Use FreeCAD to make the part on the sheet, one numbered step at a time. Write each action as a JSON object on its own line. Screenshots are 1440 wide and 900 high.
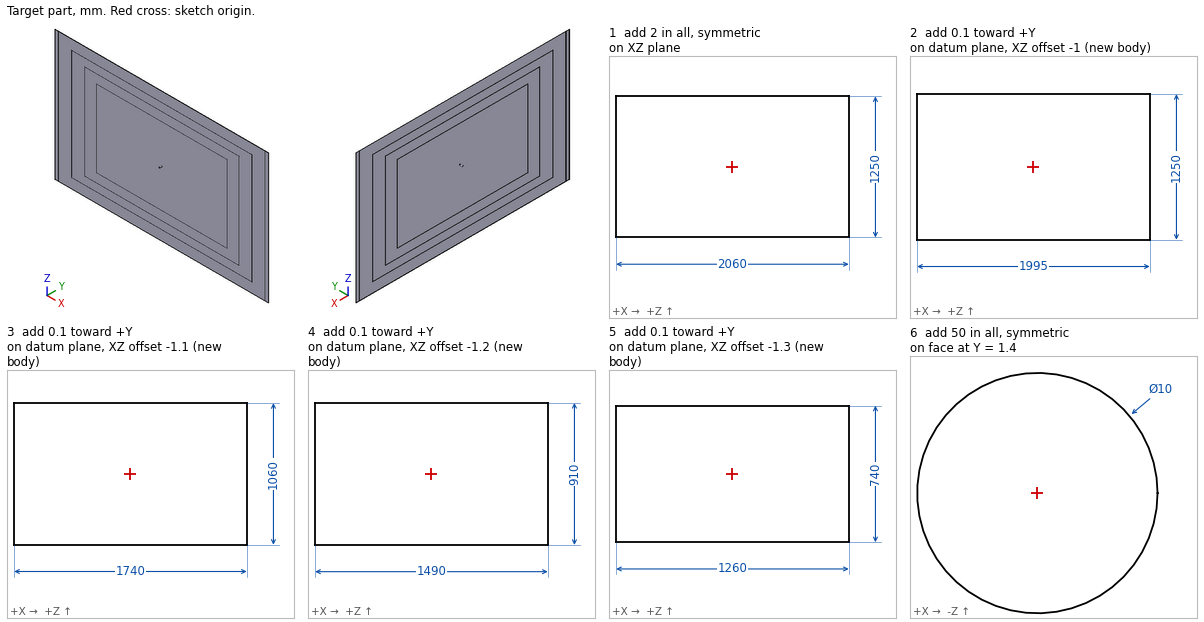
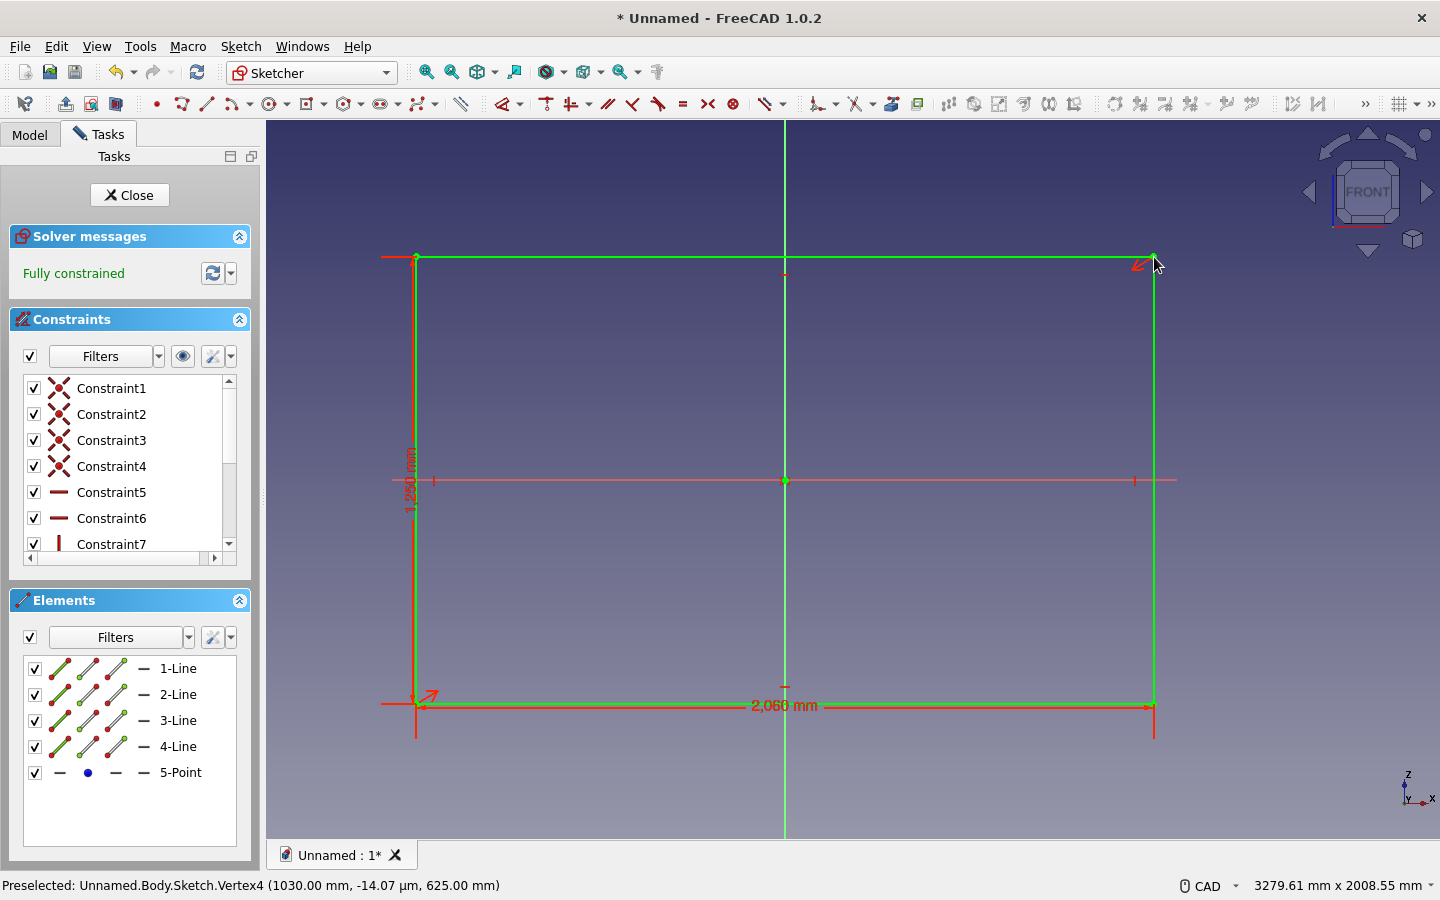
{"action": "left_click", "coordinate": [130, 195]}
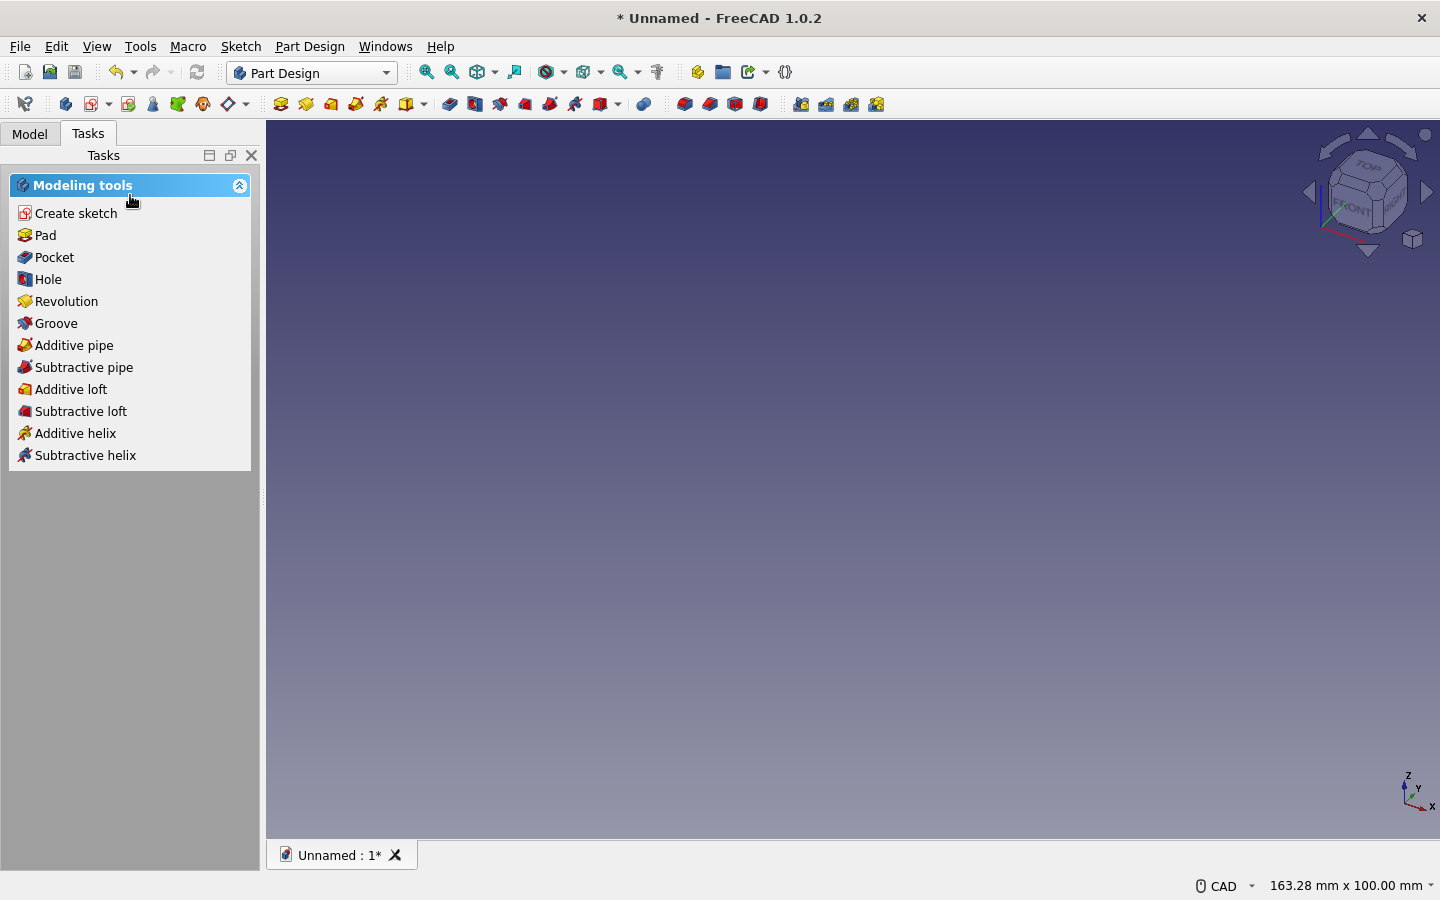
{"action": "left_click", "coordinate": [281, 104]}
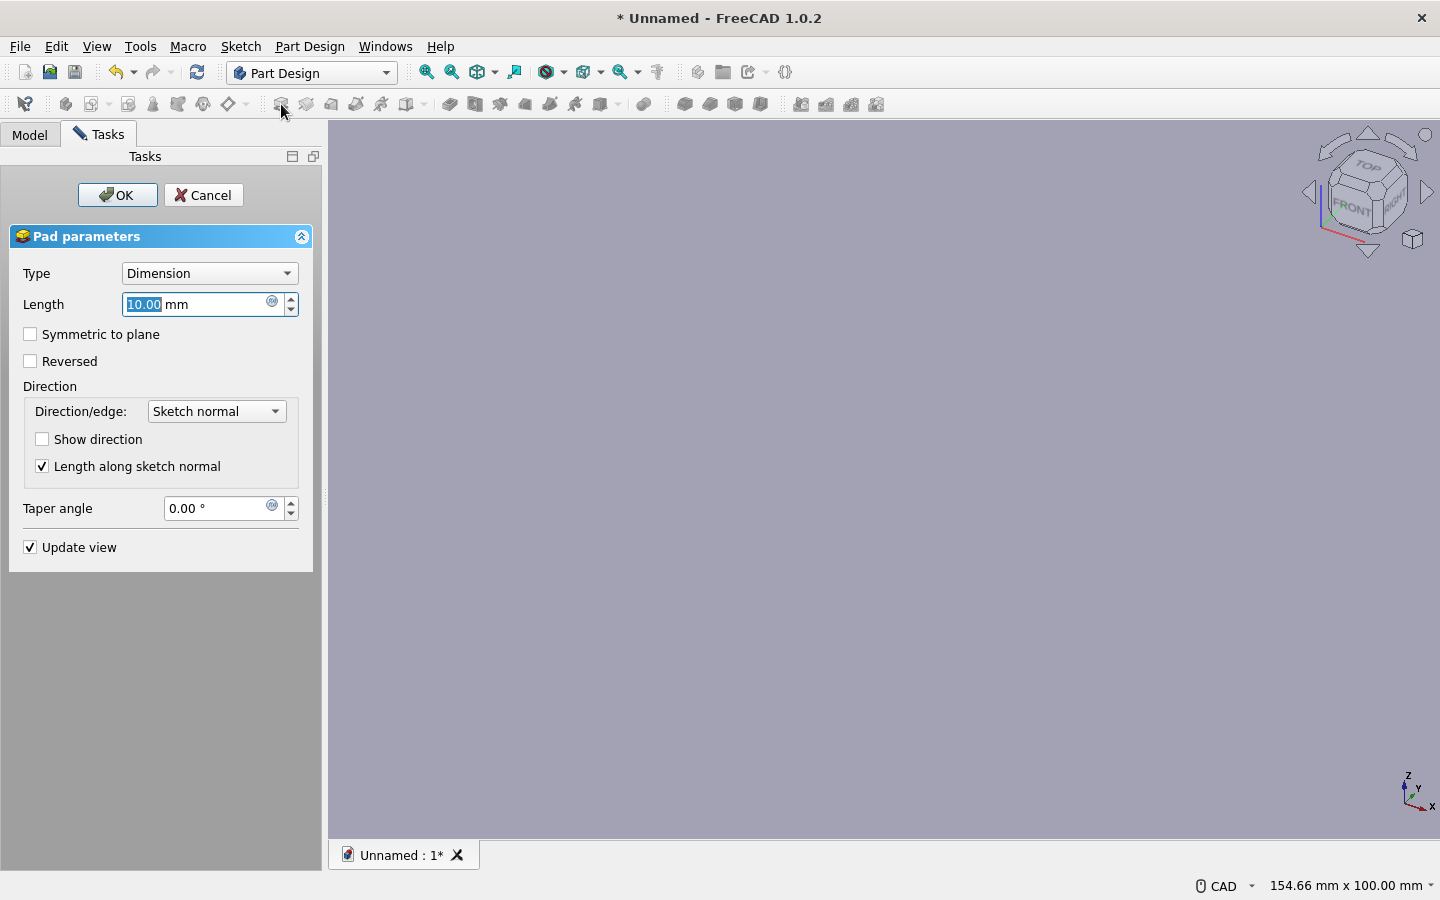
{"action": "type", "text": "2"}
{"action": "key", "text": "Tab"}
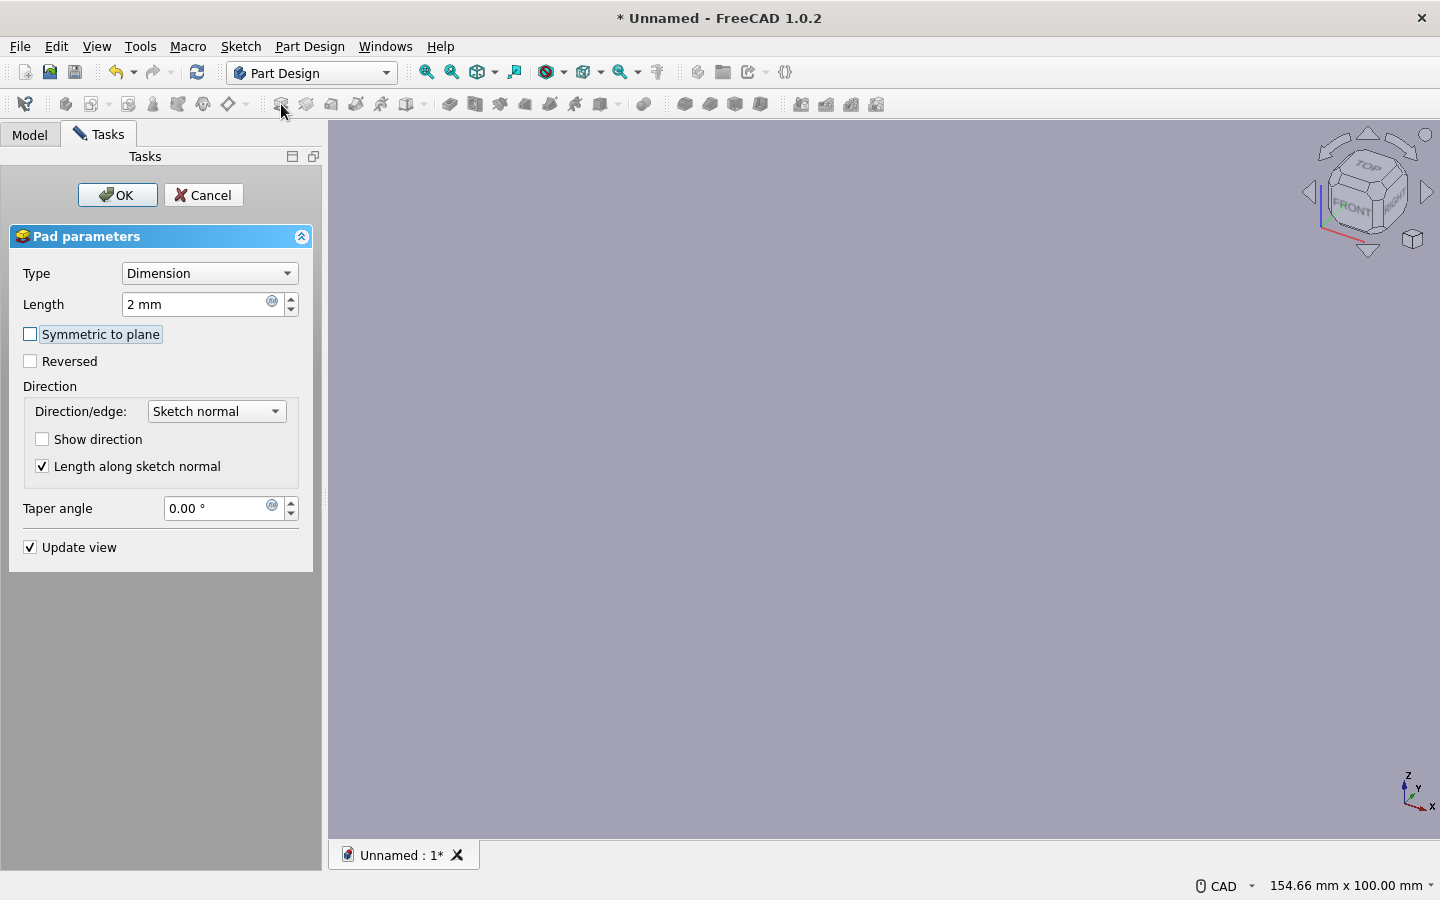
{"action": "left_click", "coordinate": [31, 334]}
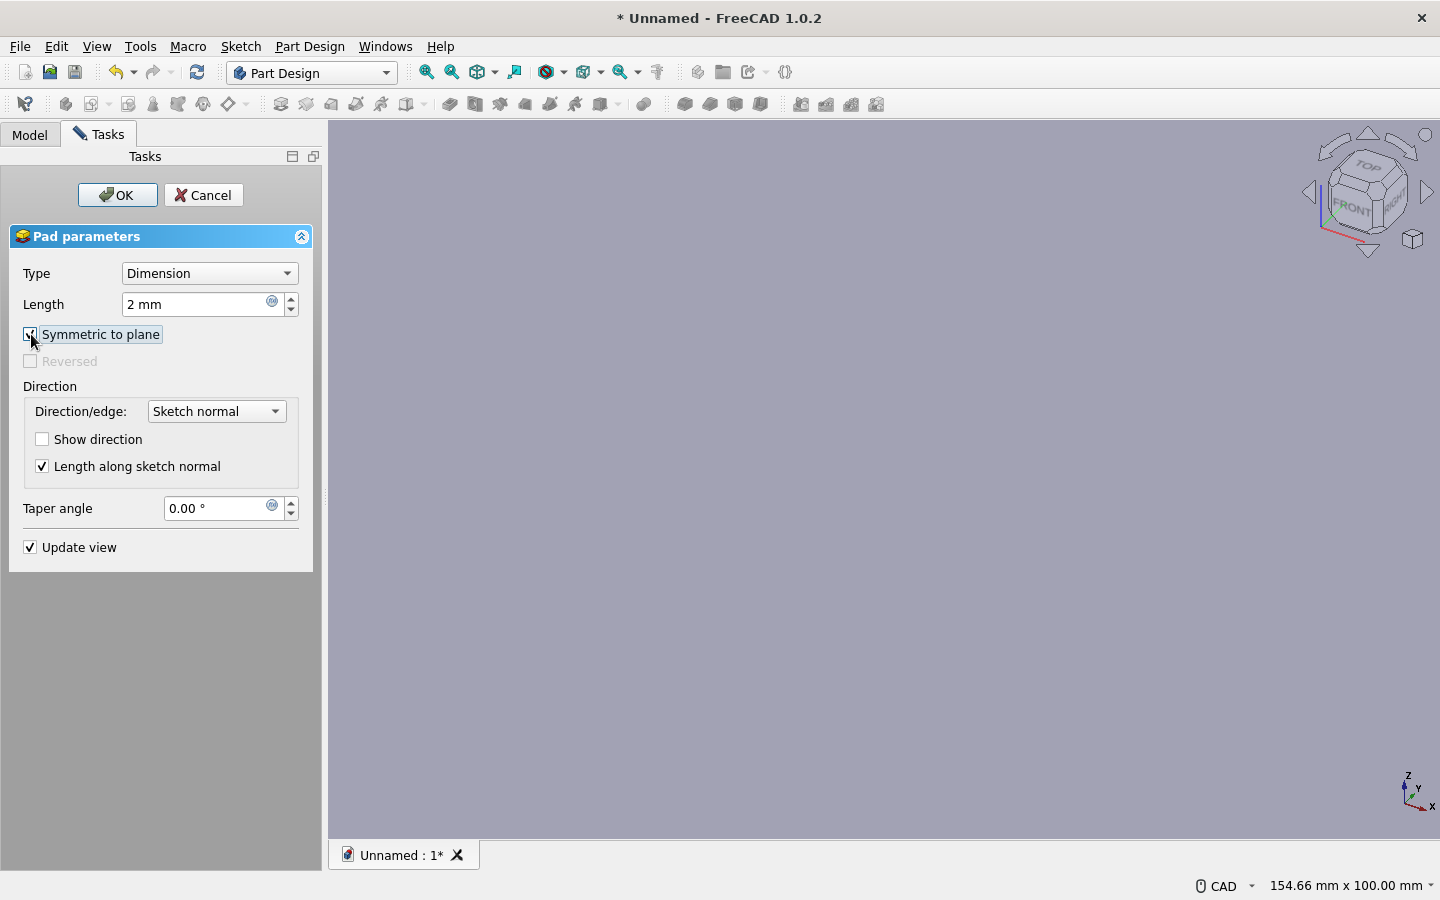
{"action": "left_click", "coordinate": [118, 195]}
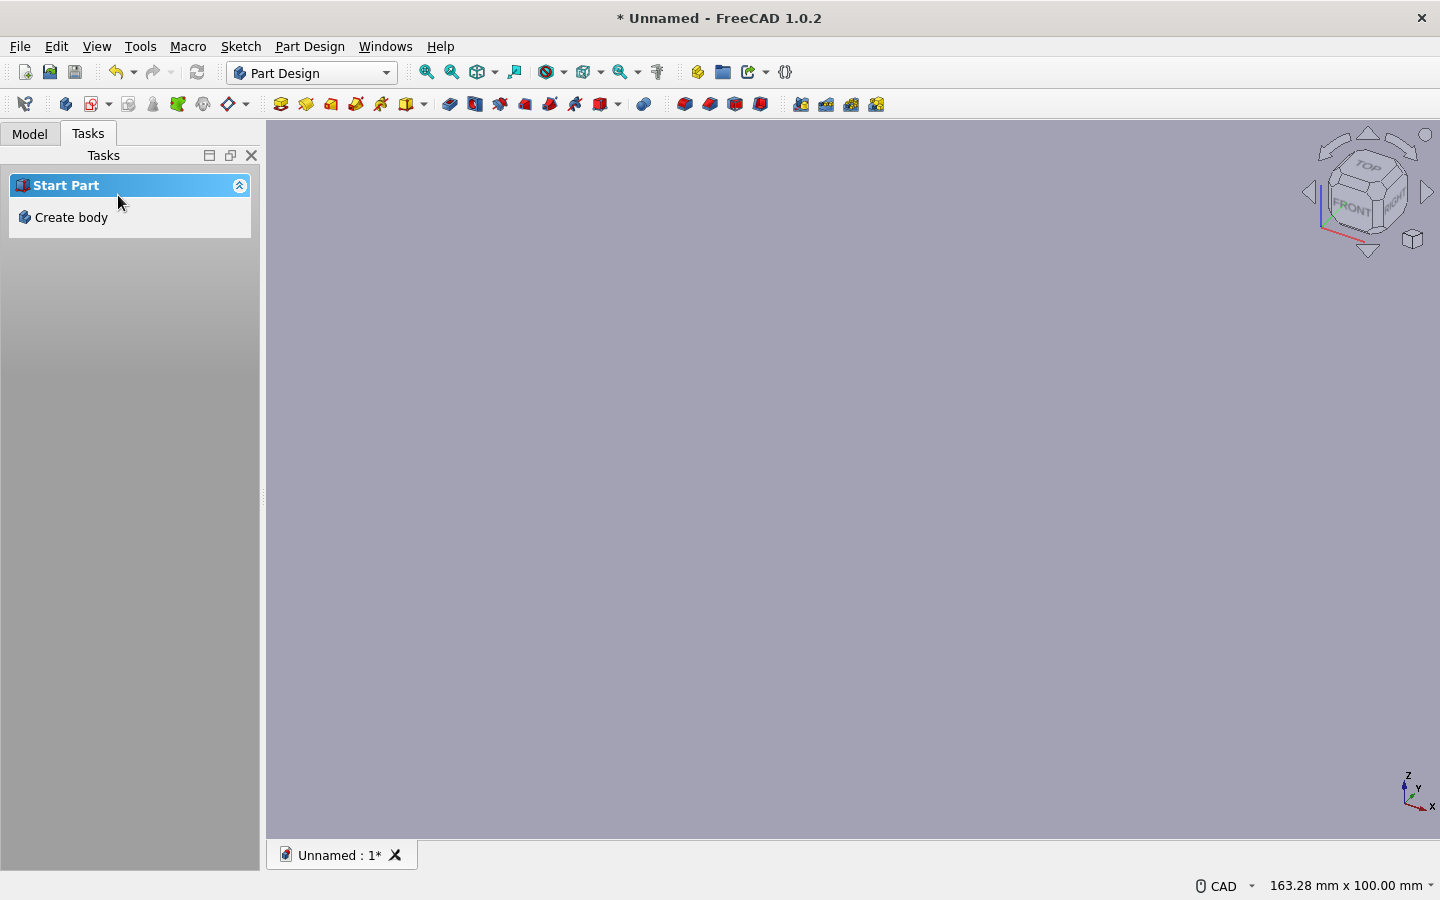
{"action": "left_click", "coordinate": [427, 72]}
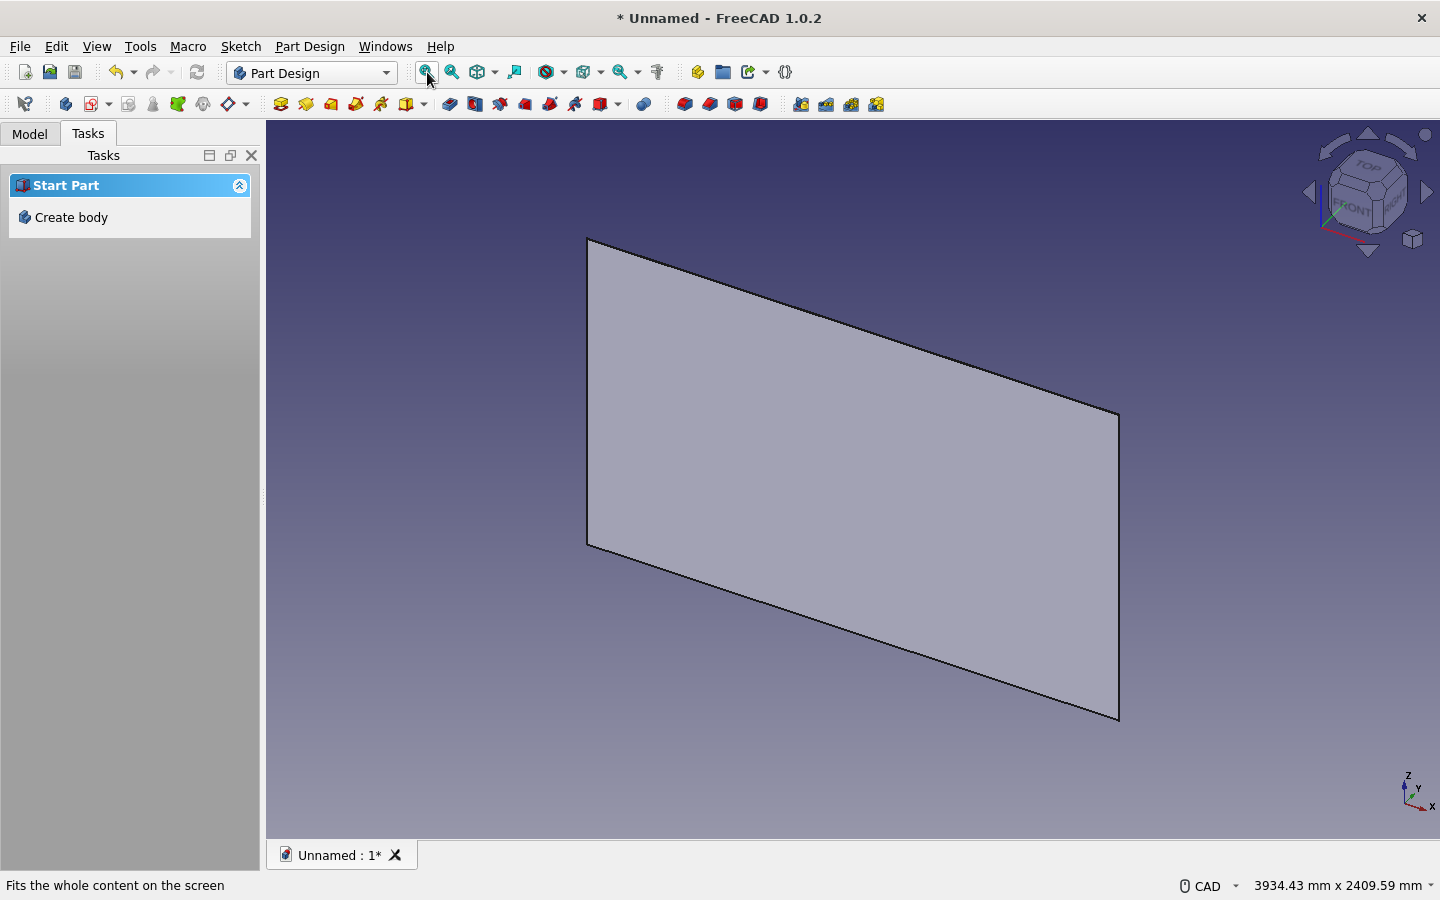
{"action": "left_click", "coordinate": [66, 104]}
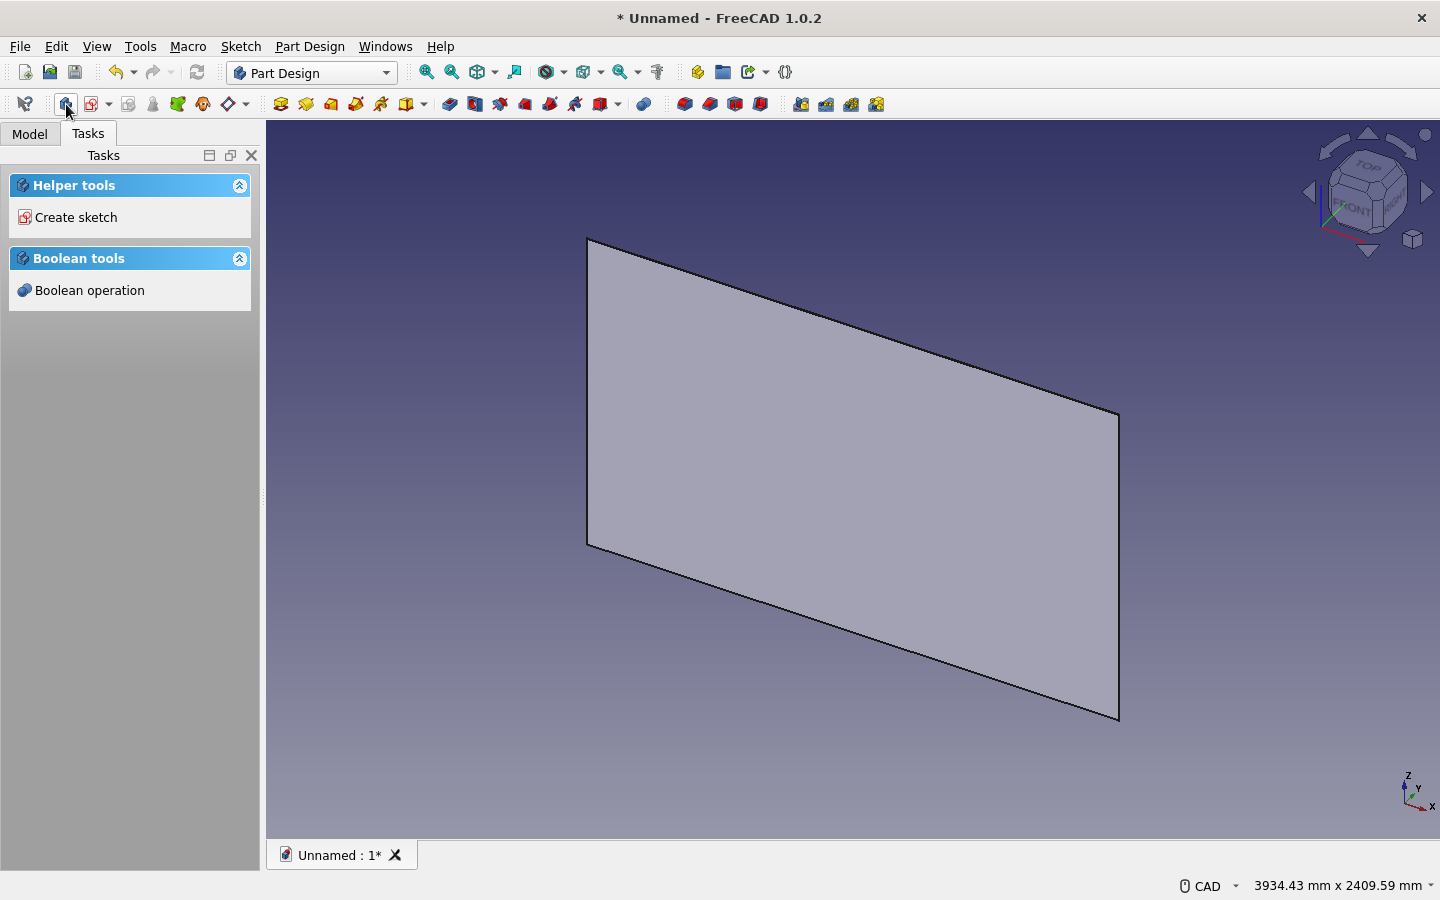
{"action": "left_click", "coordinate": [30, 134]}